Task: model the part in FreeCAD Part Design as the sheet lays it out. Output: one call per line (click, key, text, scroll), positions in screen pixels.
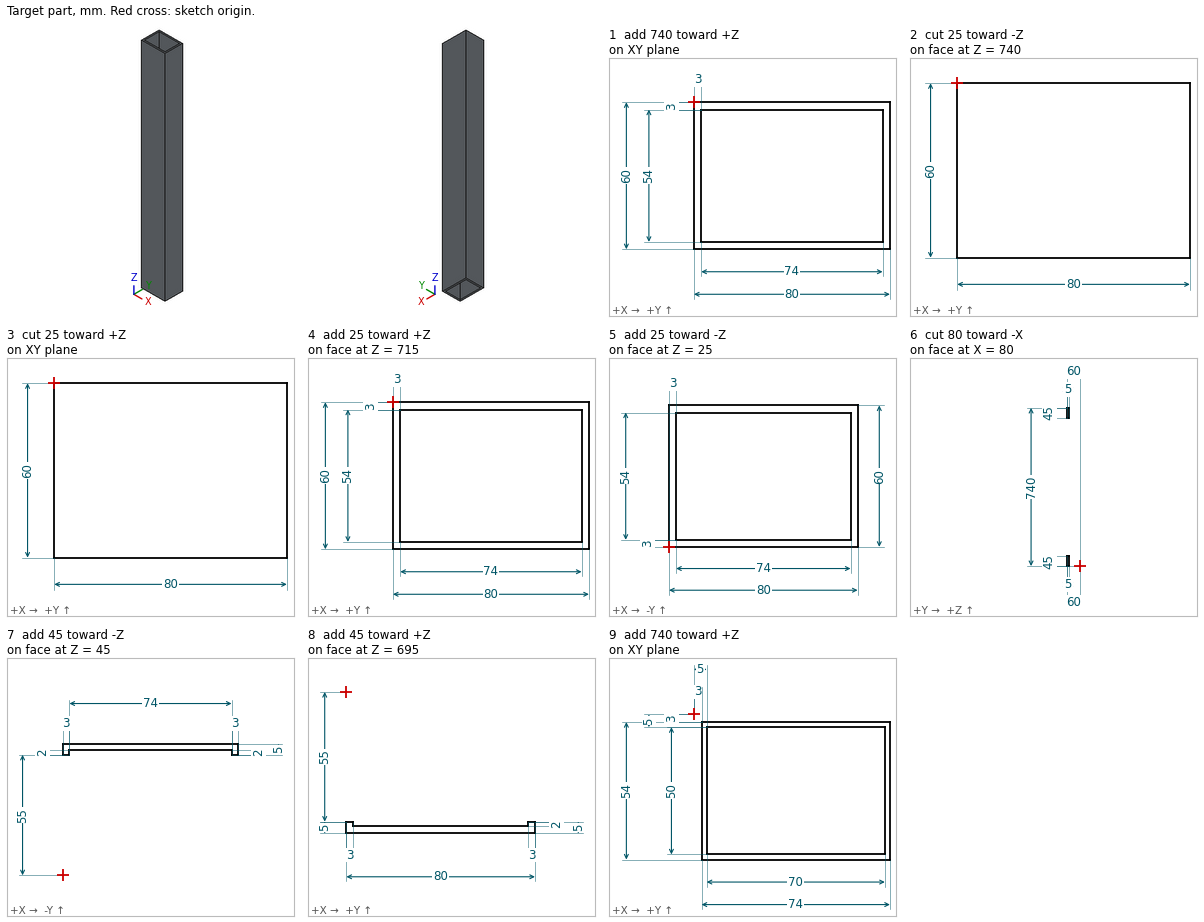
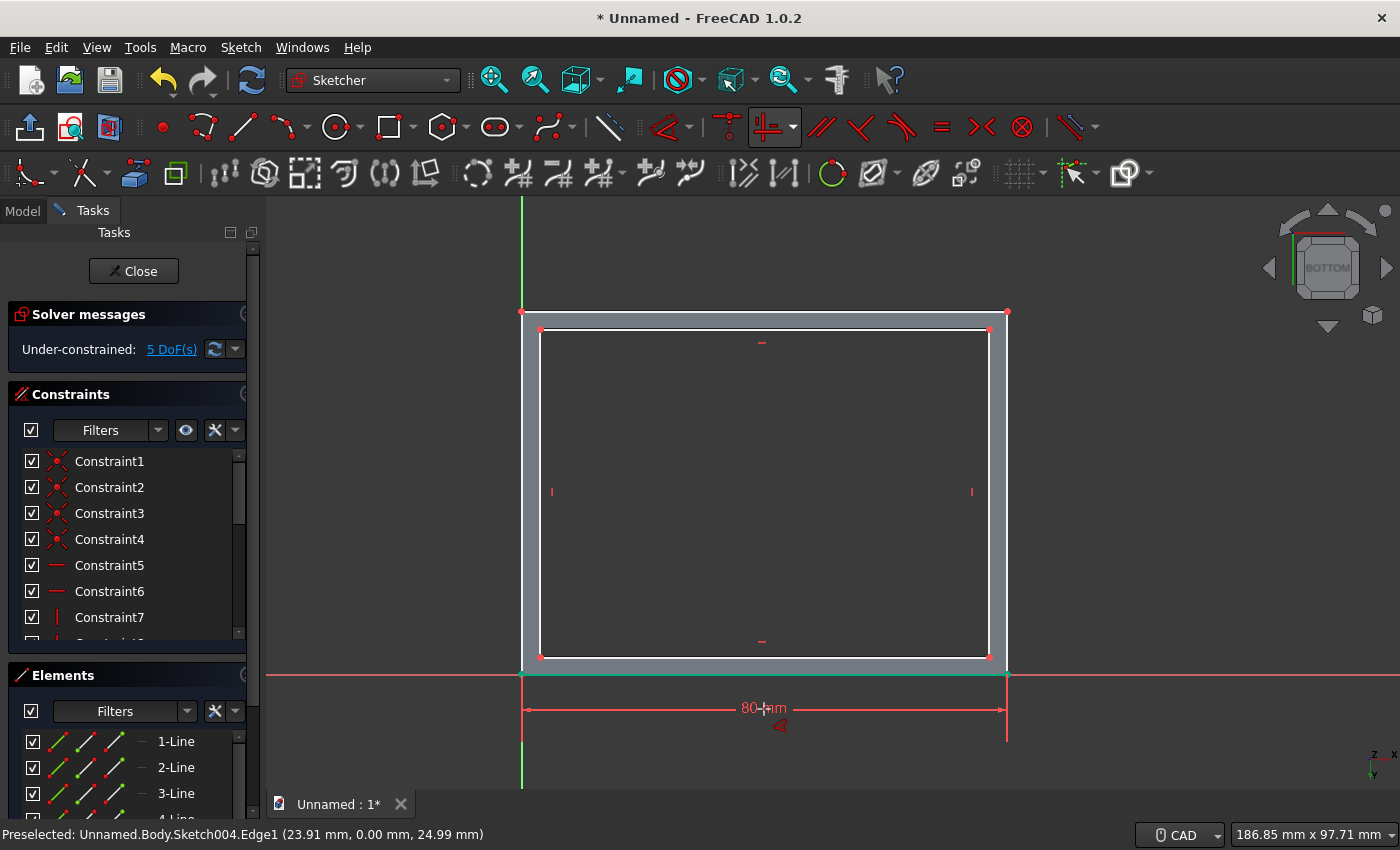
click(1007, 566)
click(1041, 493)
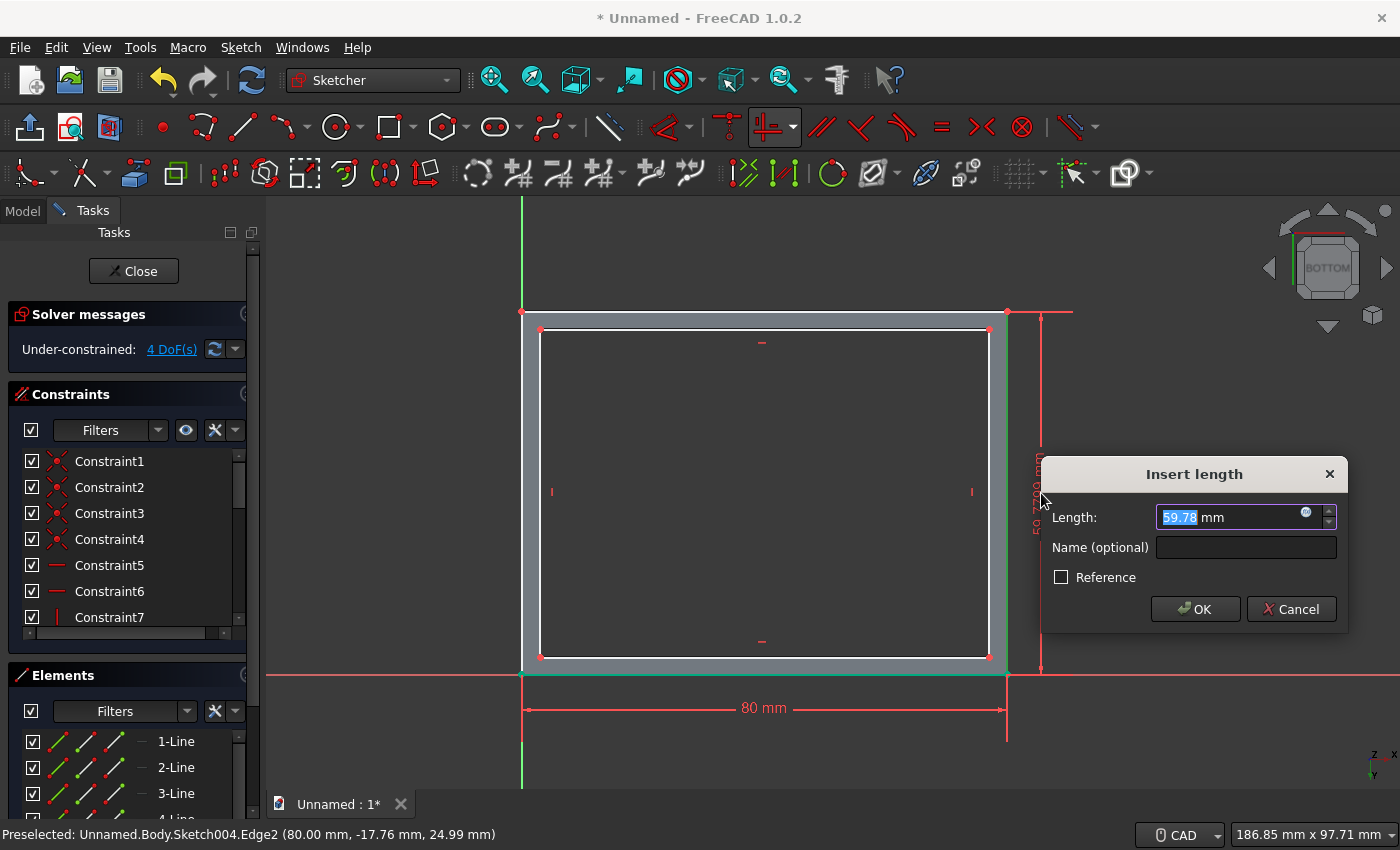
text(60)
key(Return)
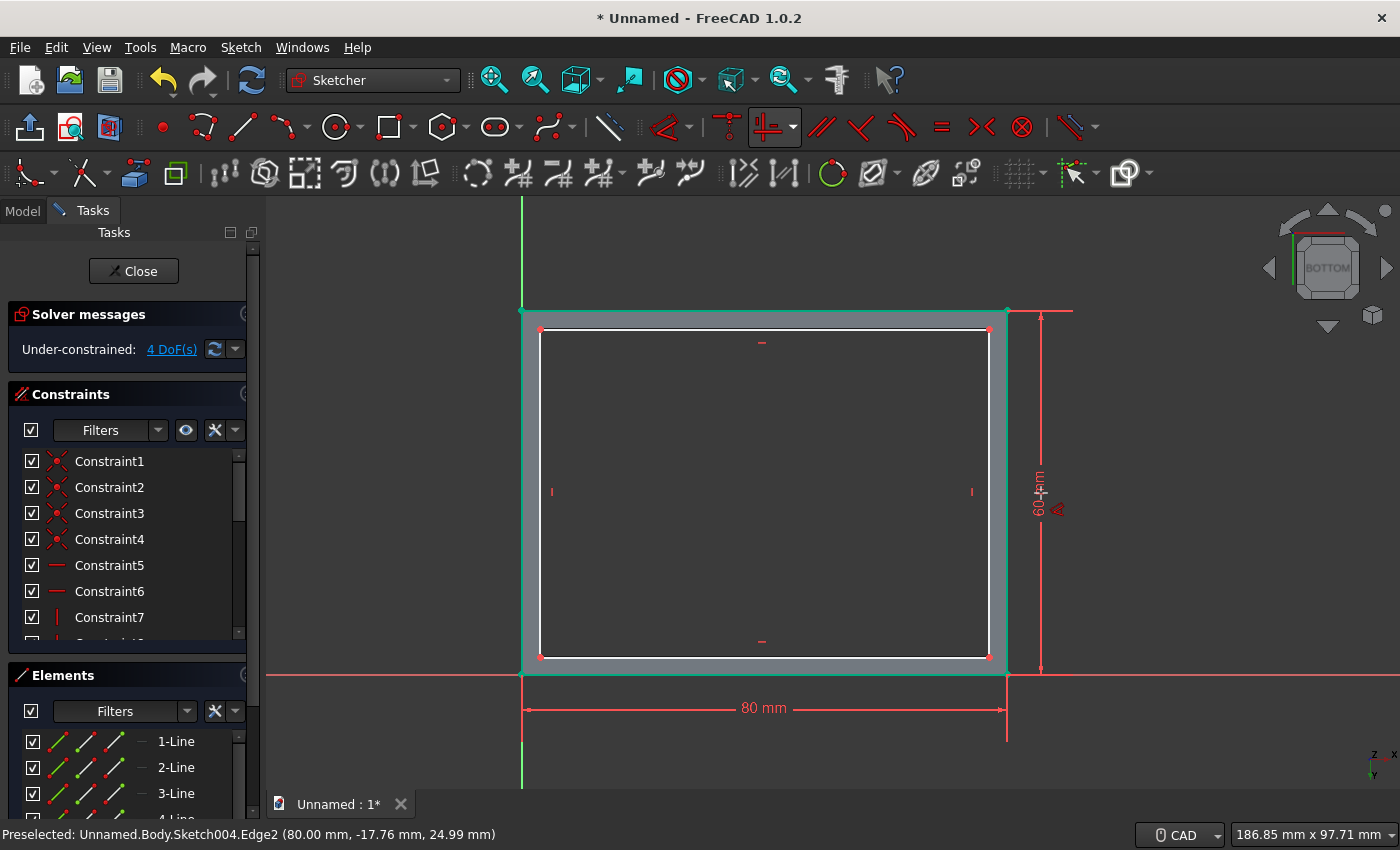
click(540, 428)
click(506, 494)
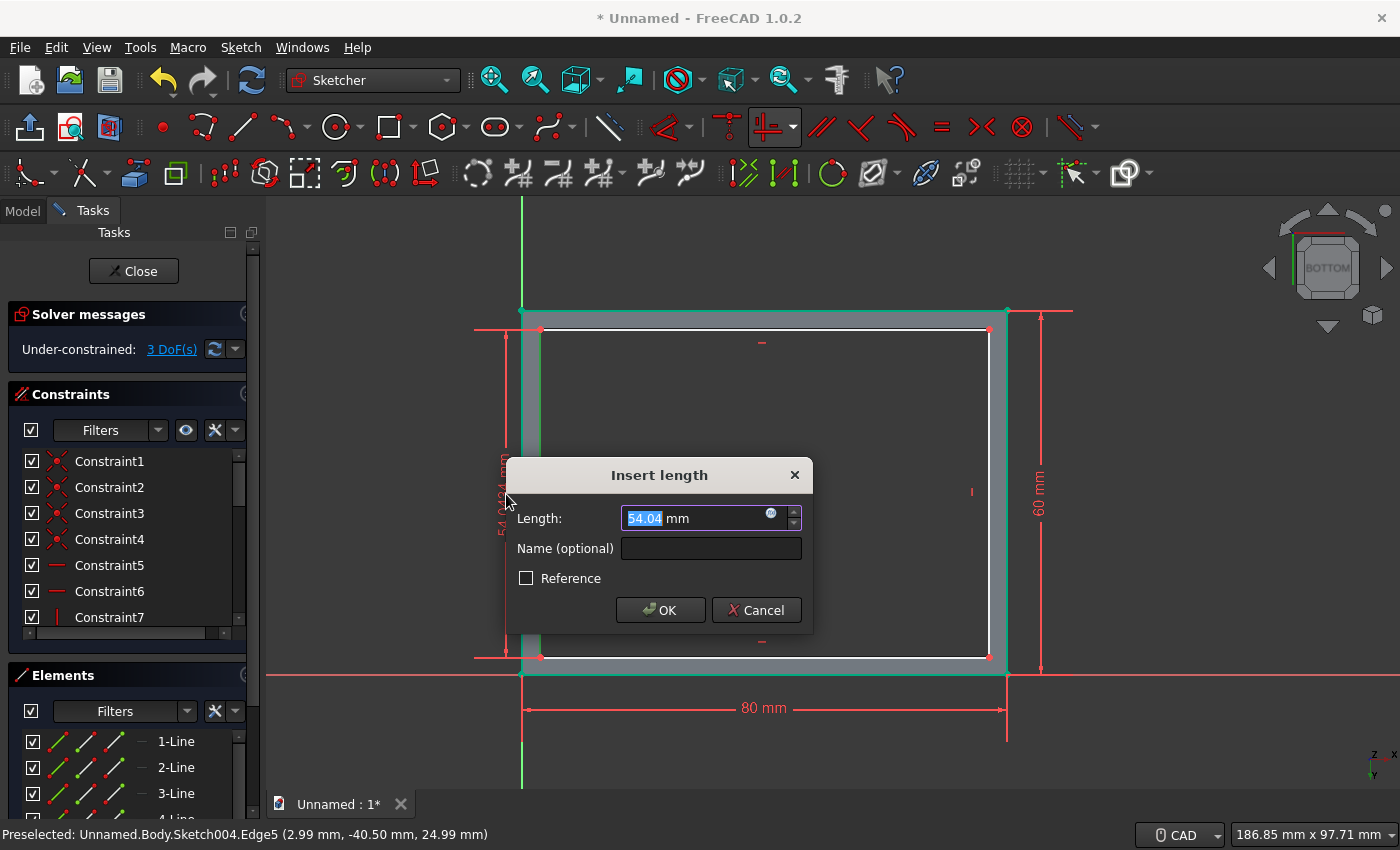
text(54)
key(Return)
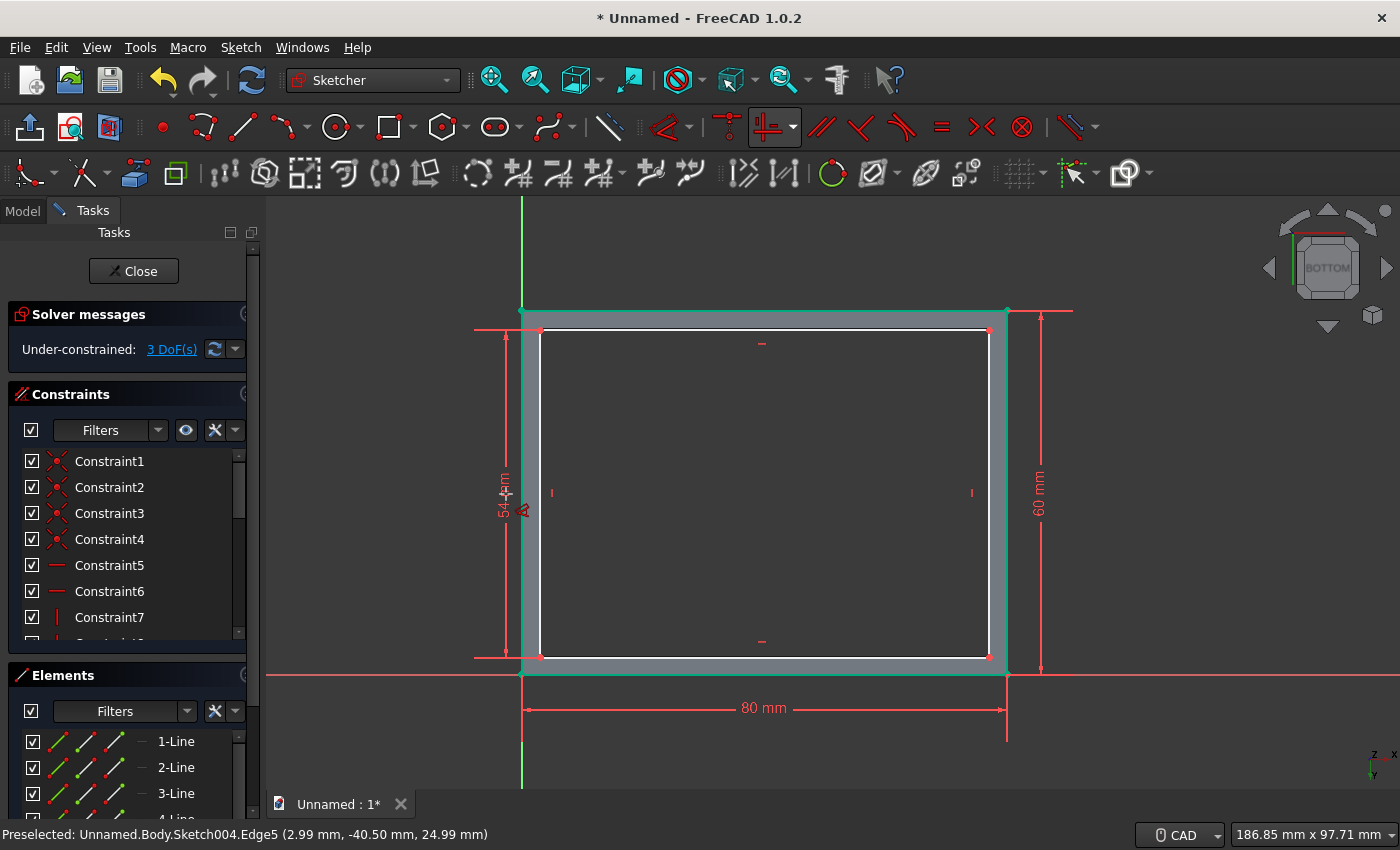
click(675, 658)
click(661, 692)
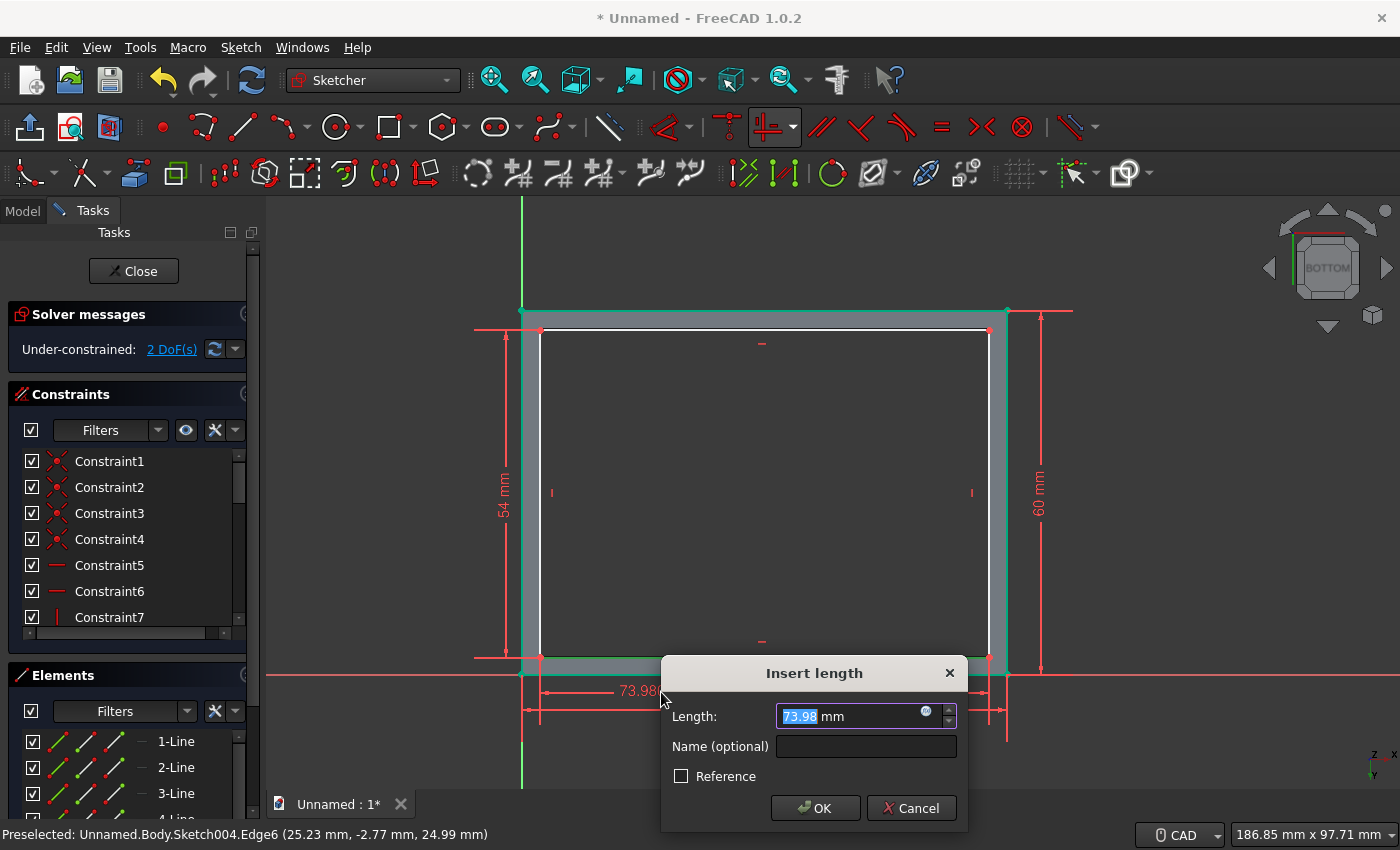
text(74)
key(Return)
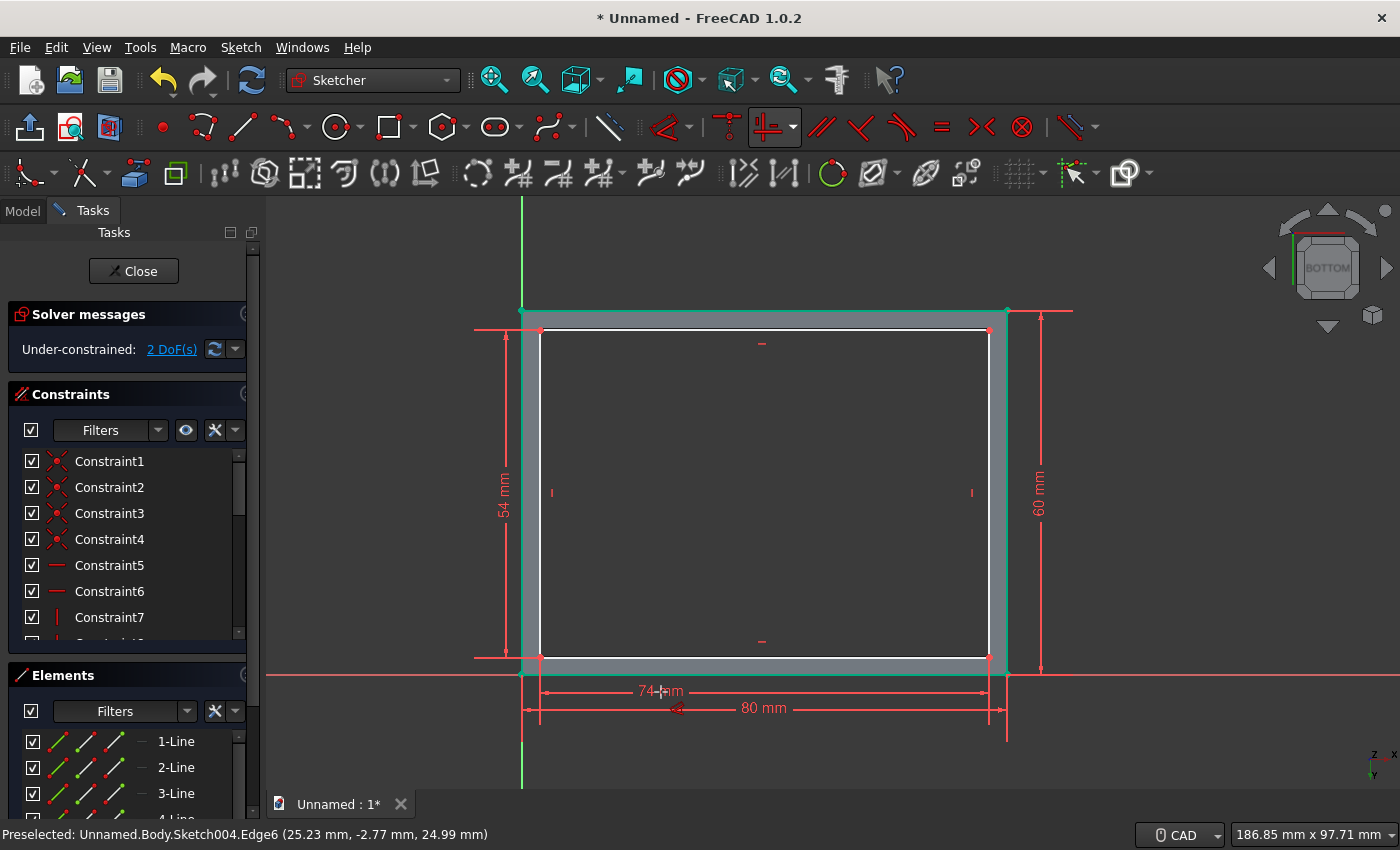
scroll(540, 330, up, 4)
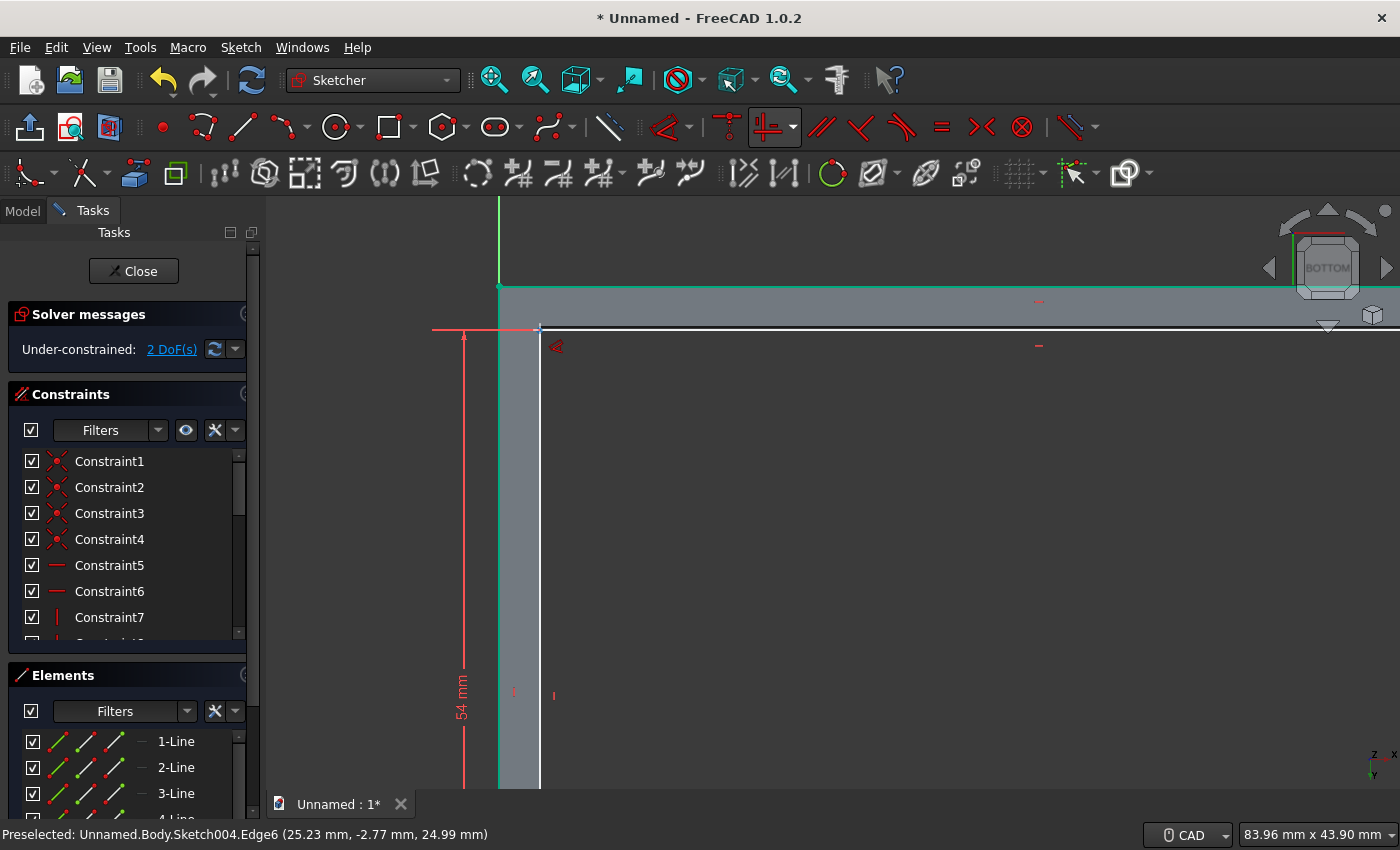
click(540, 330)
click(520, 272)